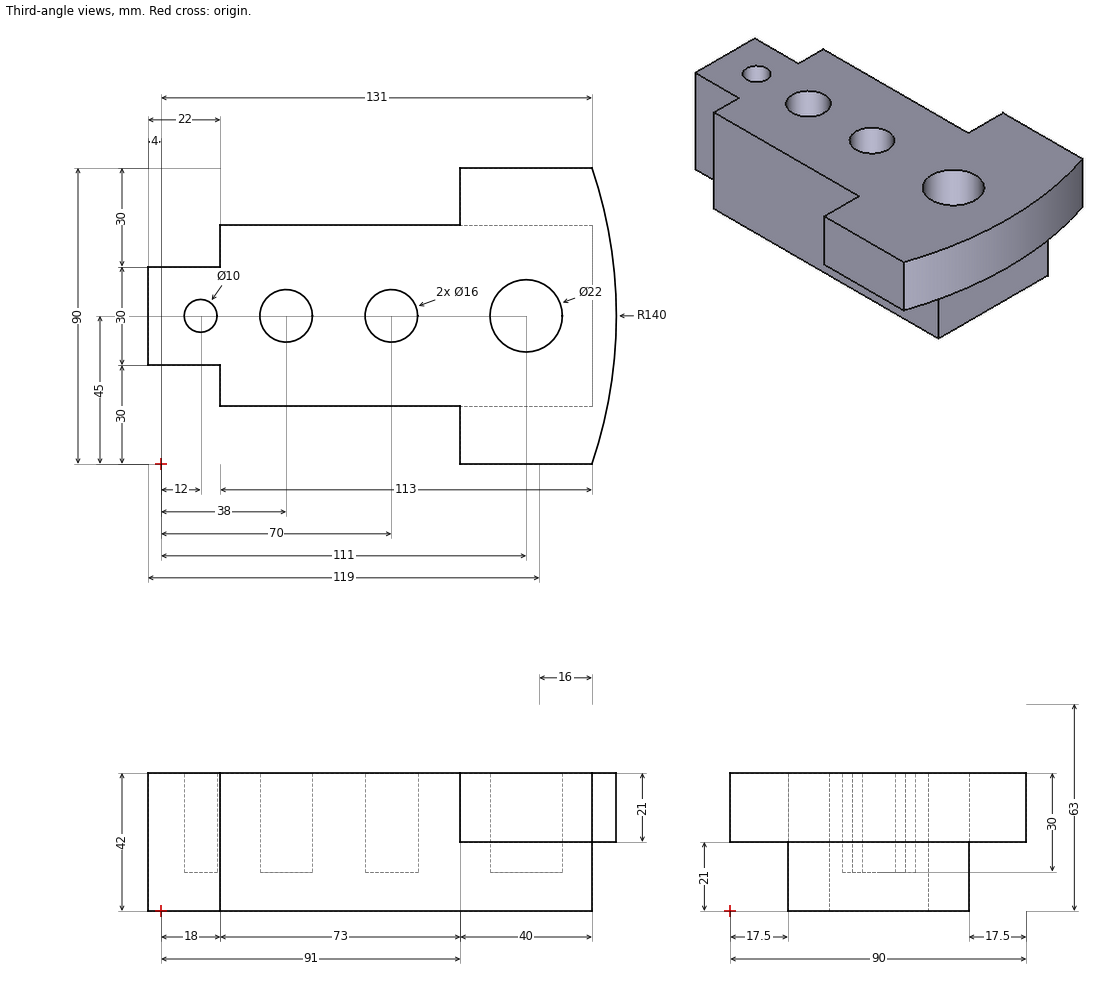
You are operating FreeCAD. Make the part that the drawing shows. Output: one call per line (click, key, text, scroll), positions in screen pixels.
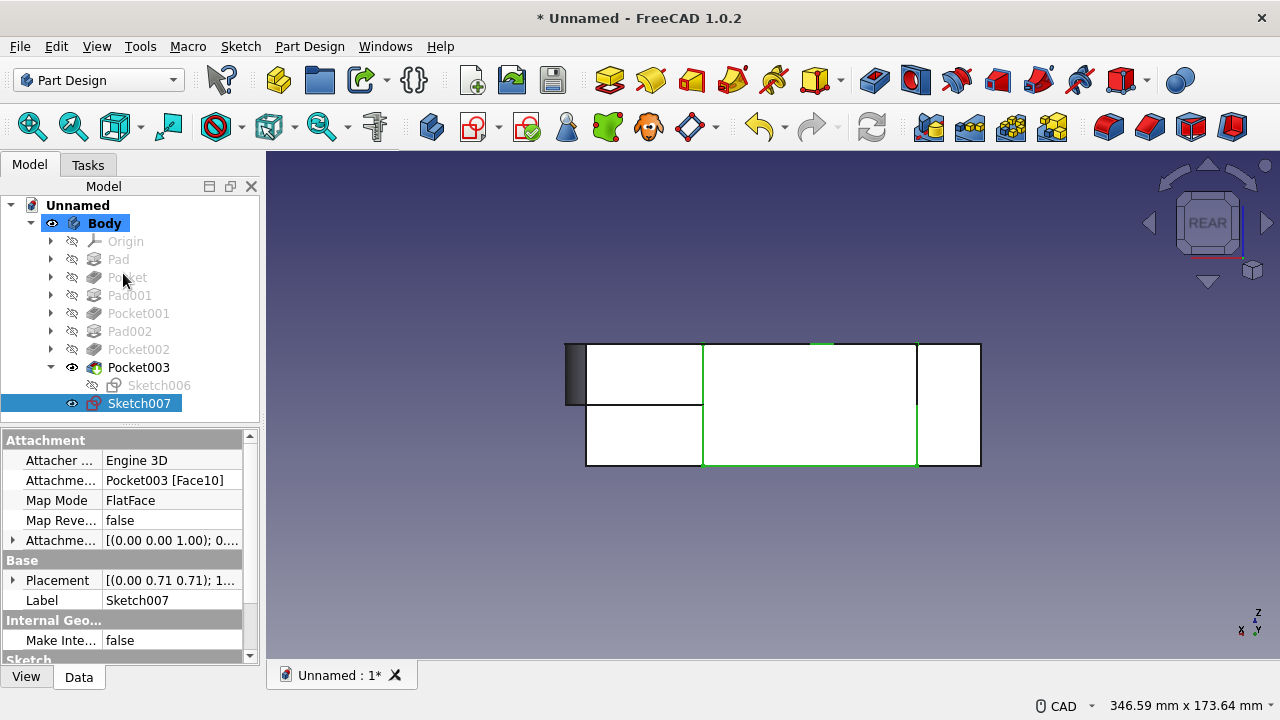
click(875, 80)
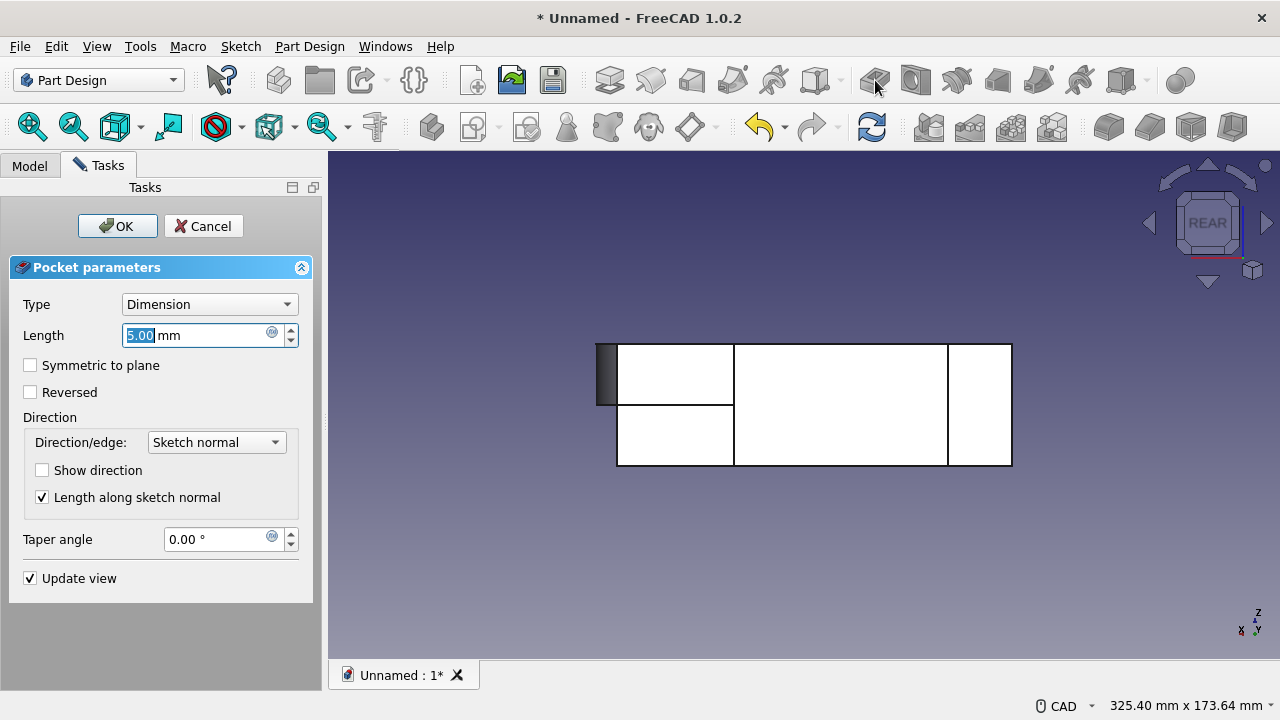
text(17.5)
key(Tab)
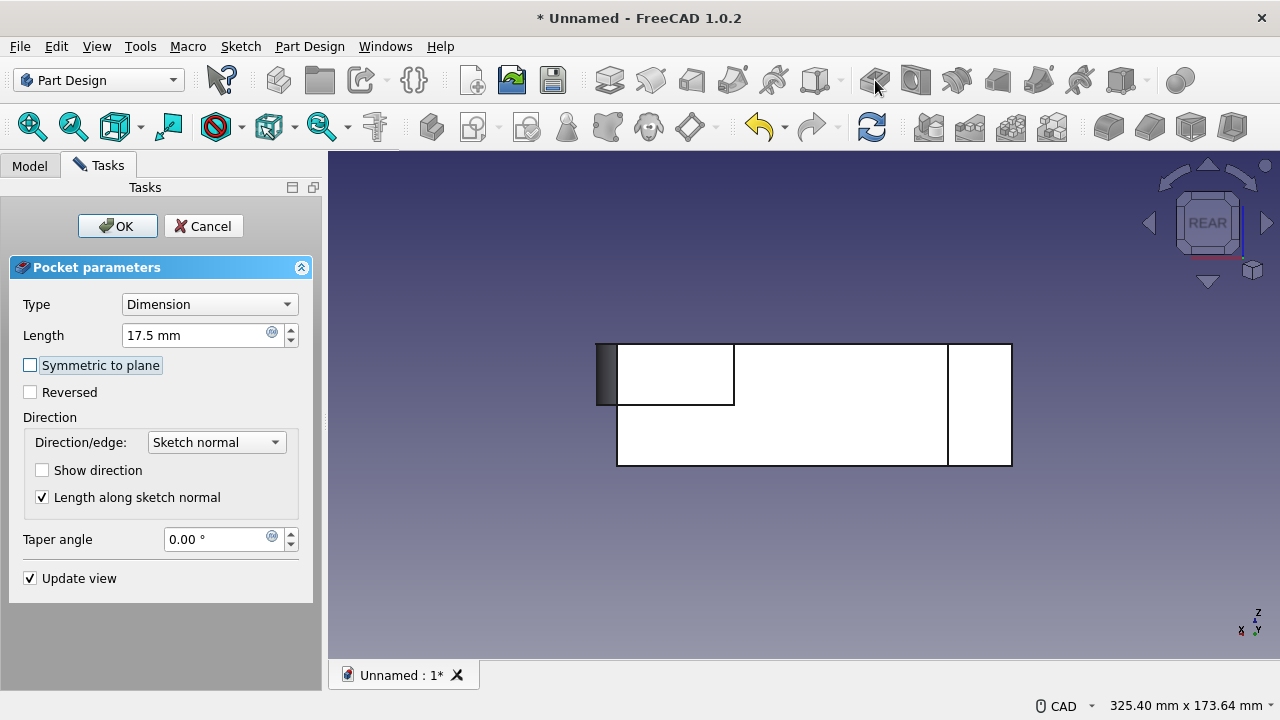
click(118, 226)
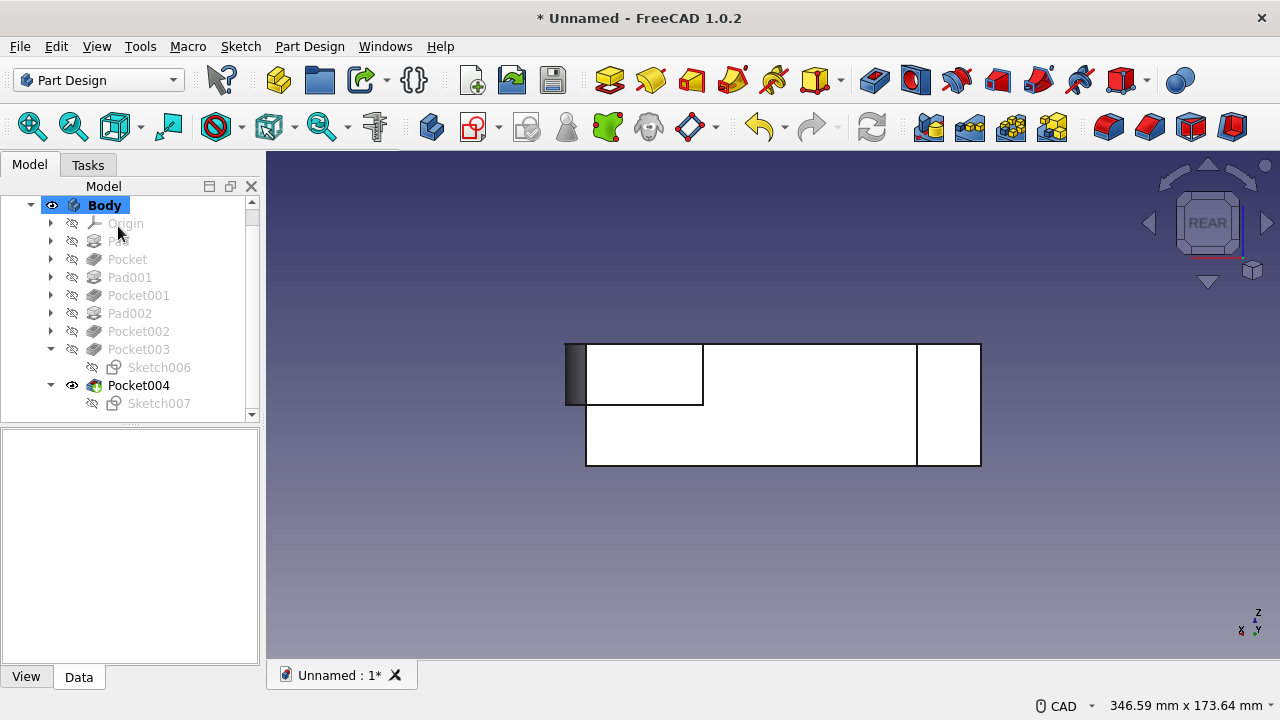
click(33, 128)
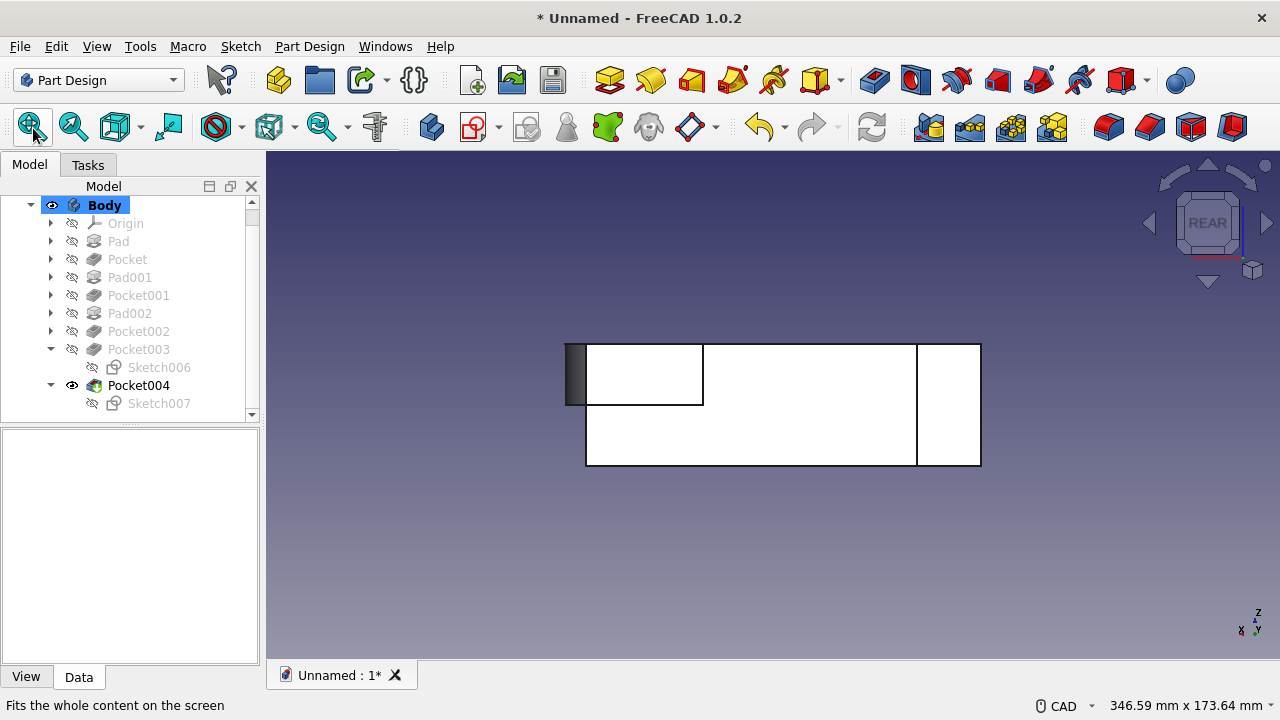
key(0)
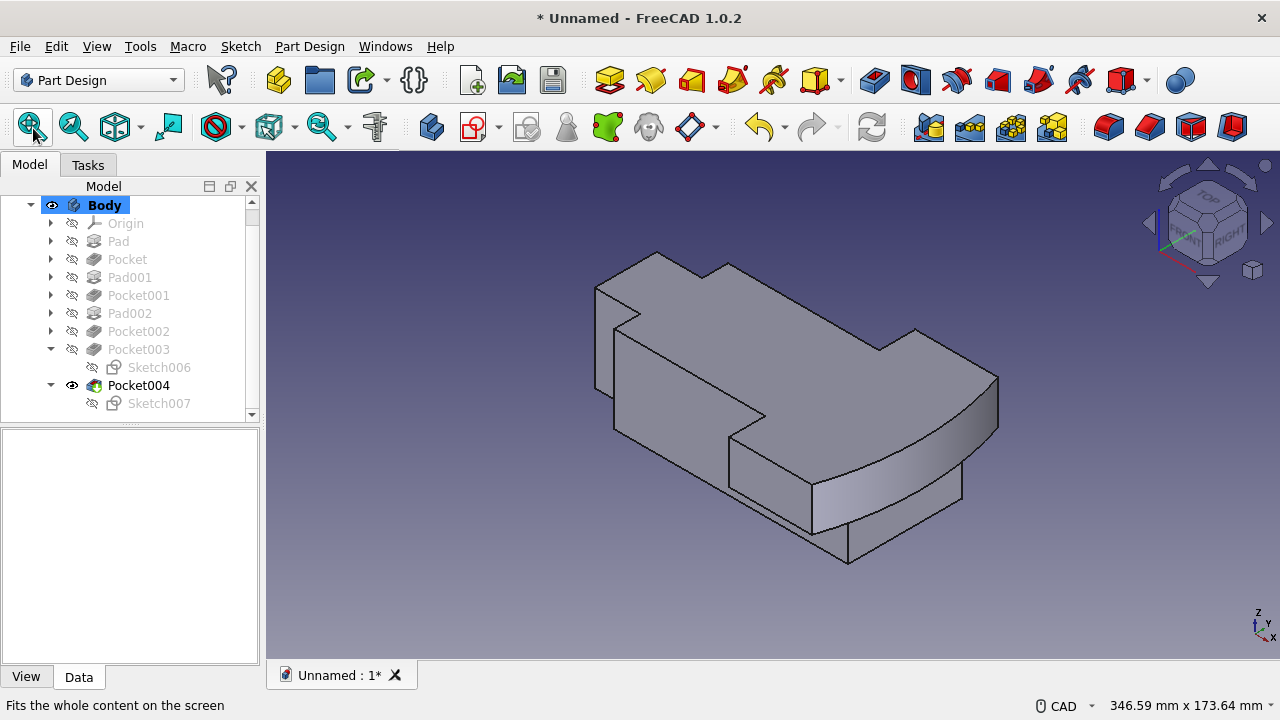
click(857, 402)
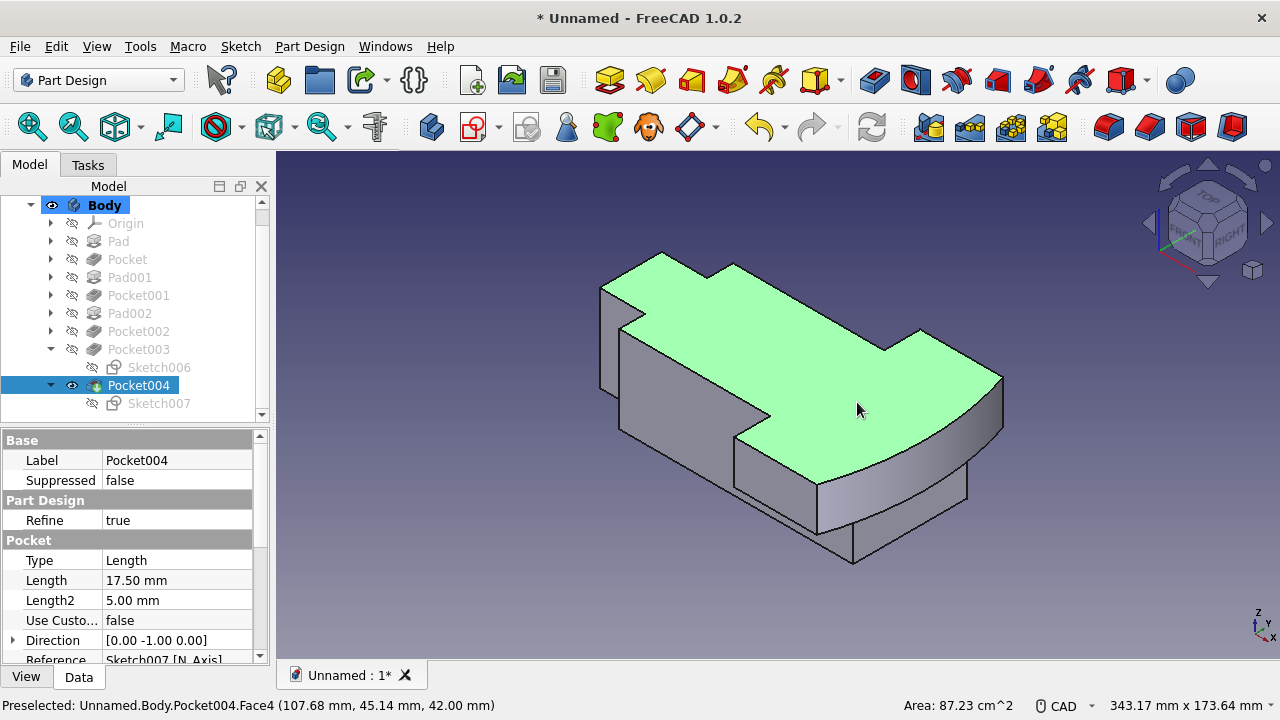
click(472, 128)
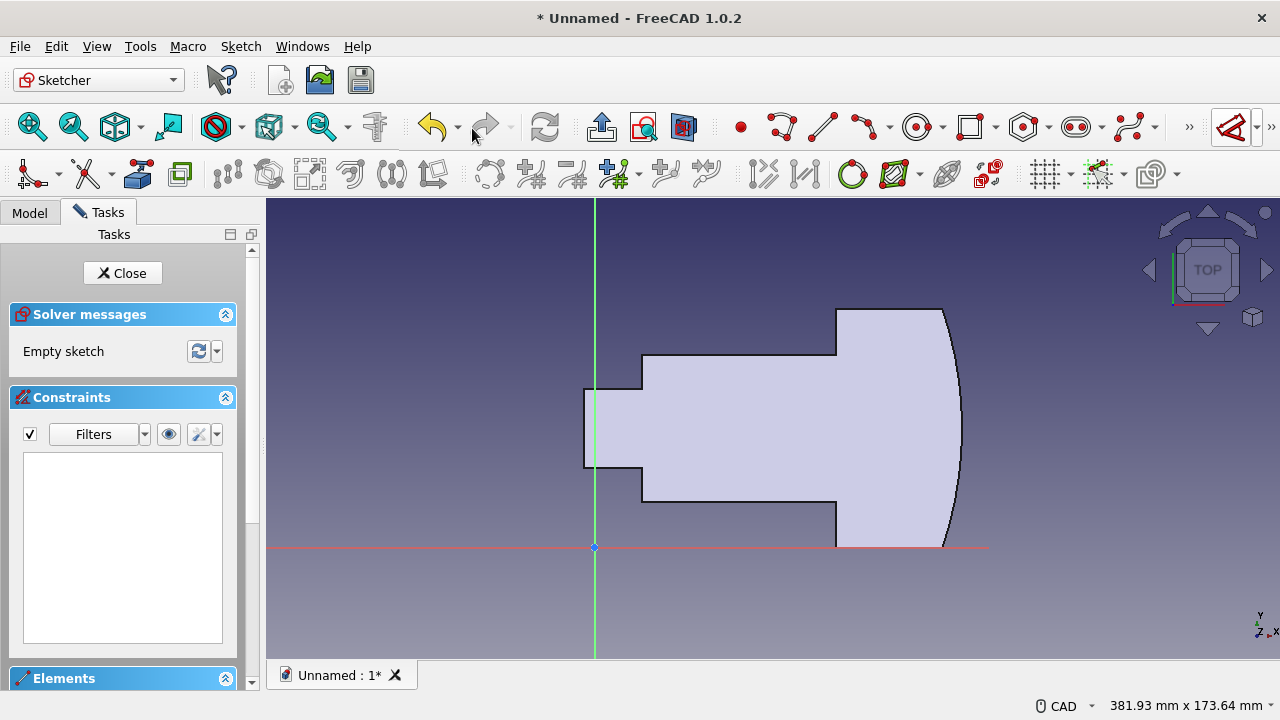
scroll(820, 529, up, 3)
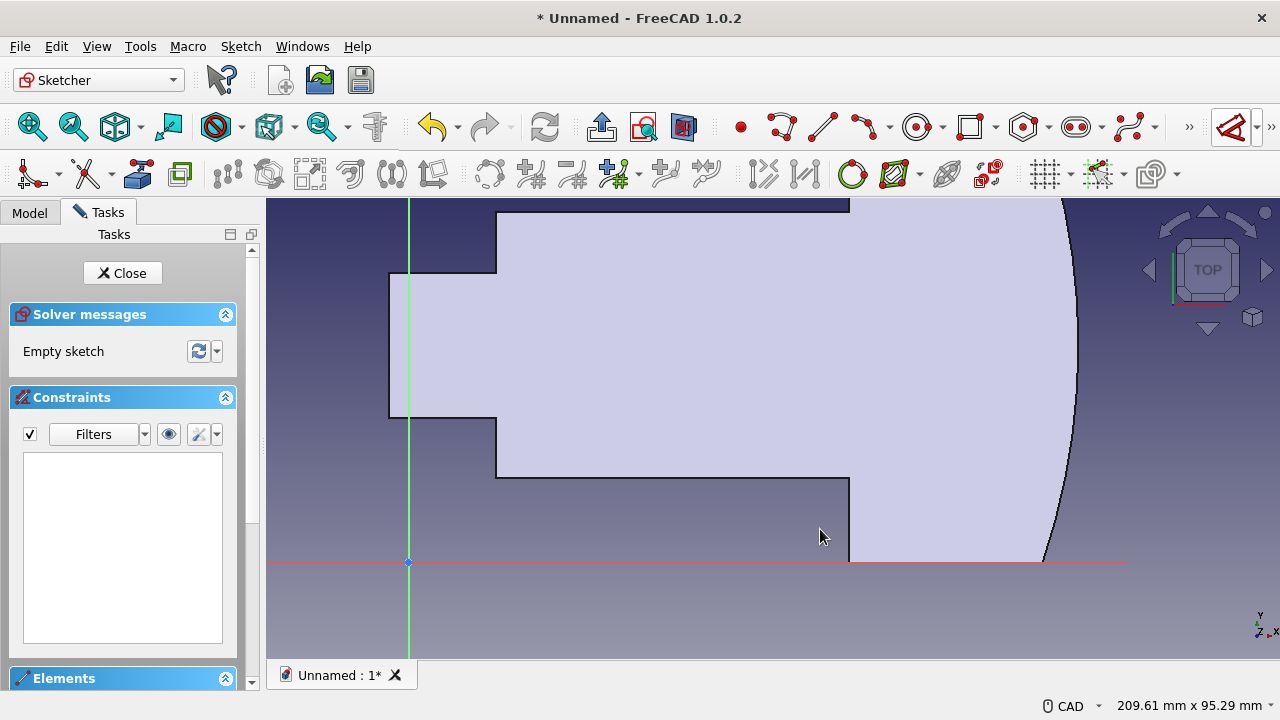
click(916, 128)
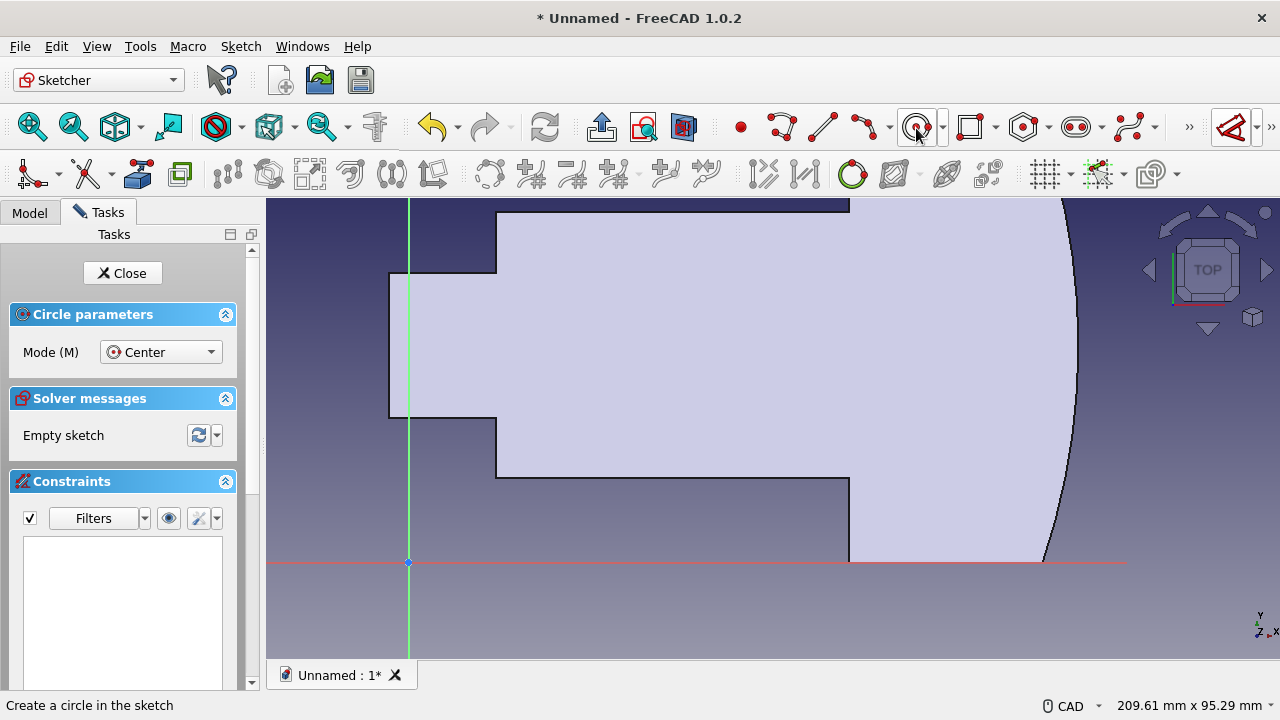
click(946, 345)
move(983, 308)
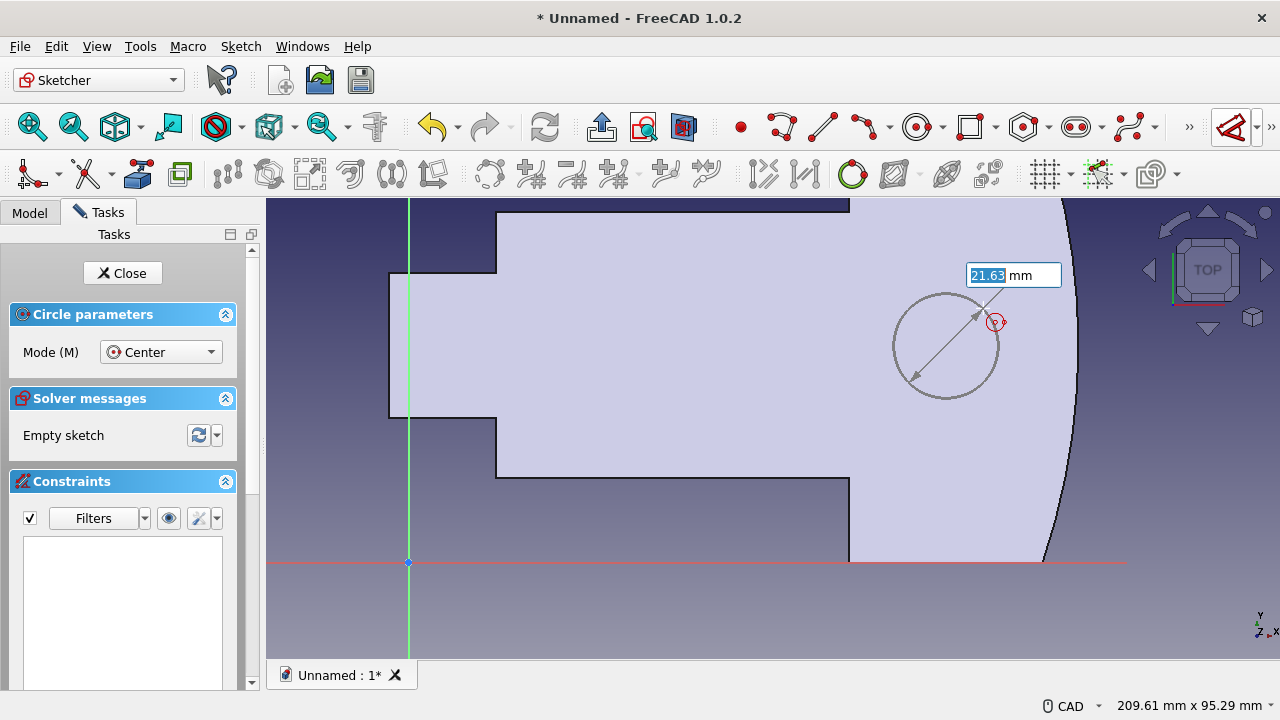
text(22)
key(Return)